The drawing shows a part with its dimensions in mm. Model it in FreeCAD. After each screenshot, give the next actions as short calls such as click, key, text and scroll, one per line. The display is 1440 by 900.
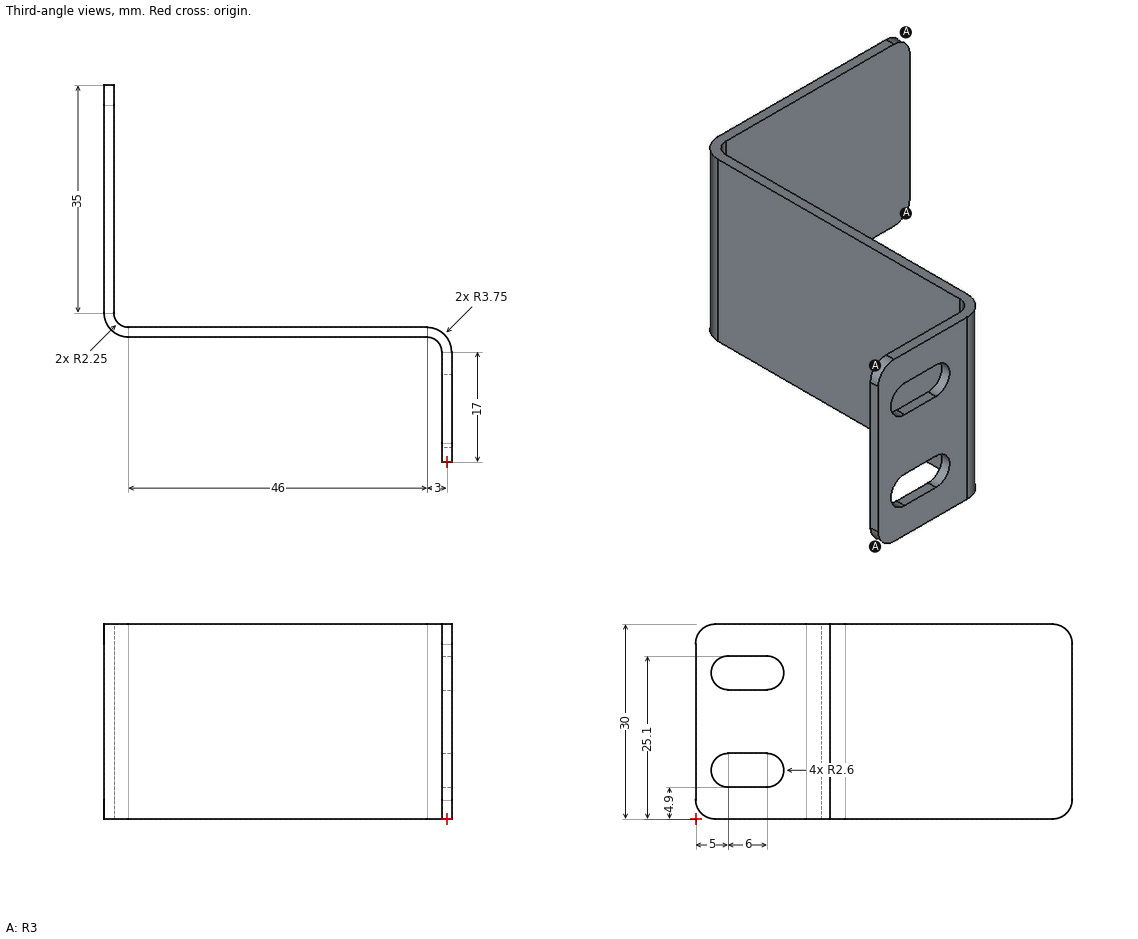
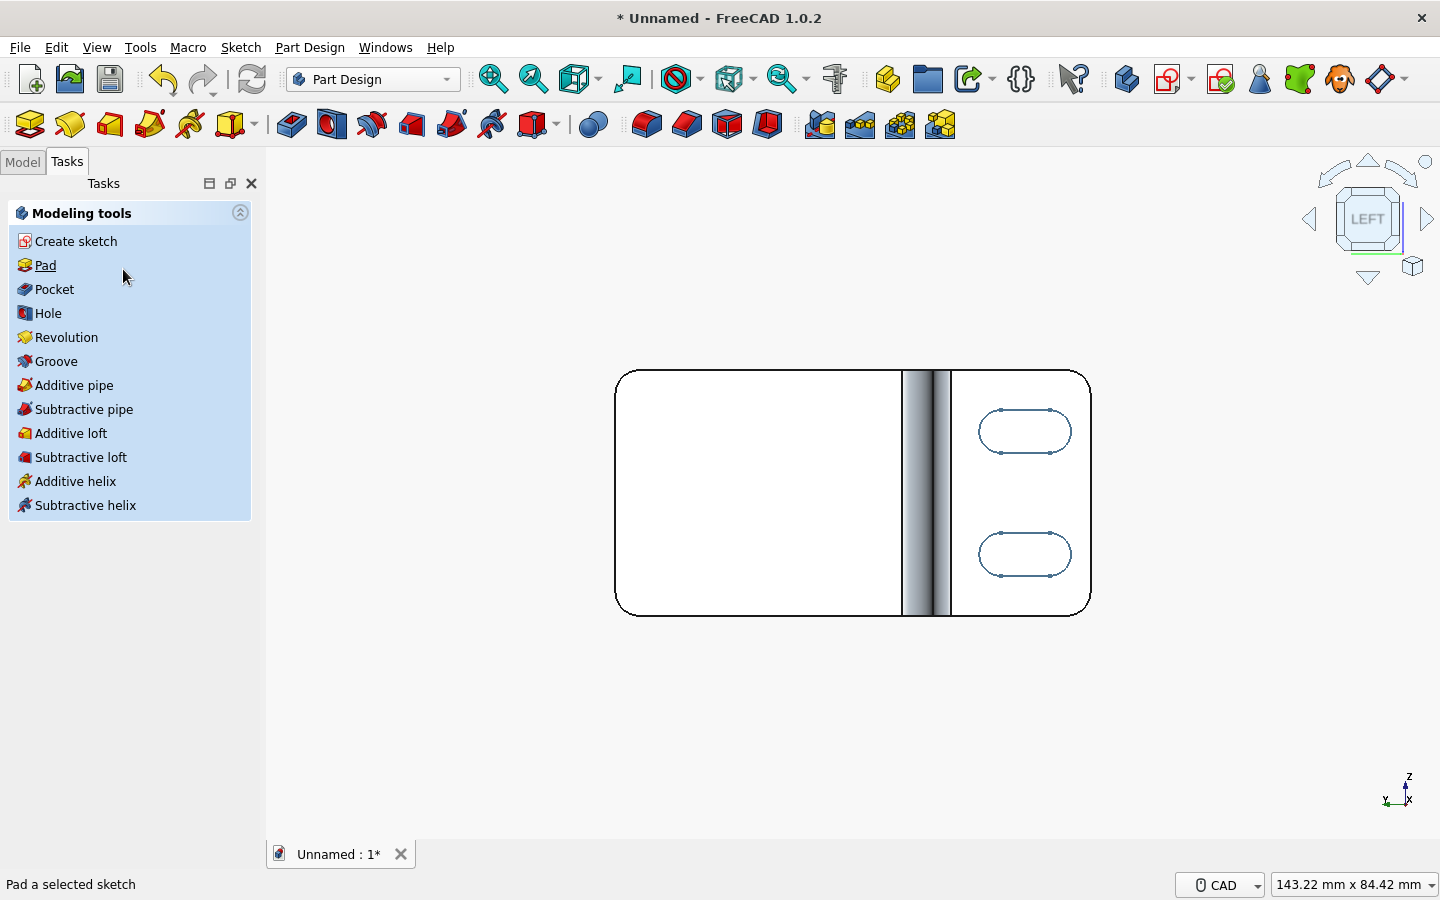
click(292, 124)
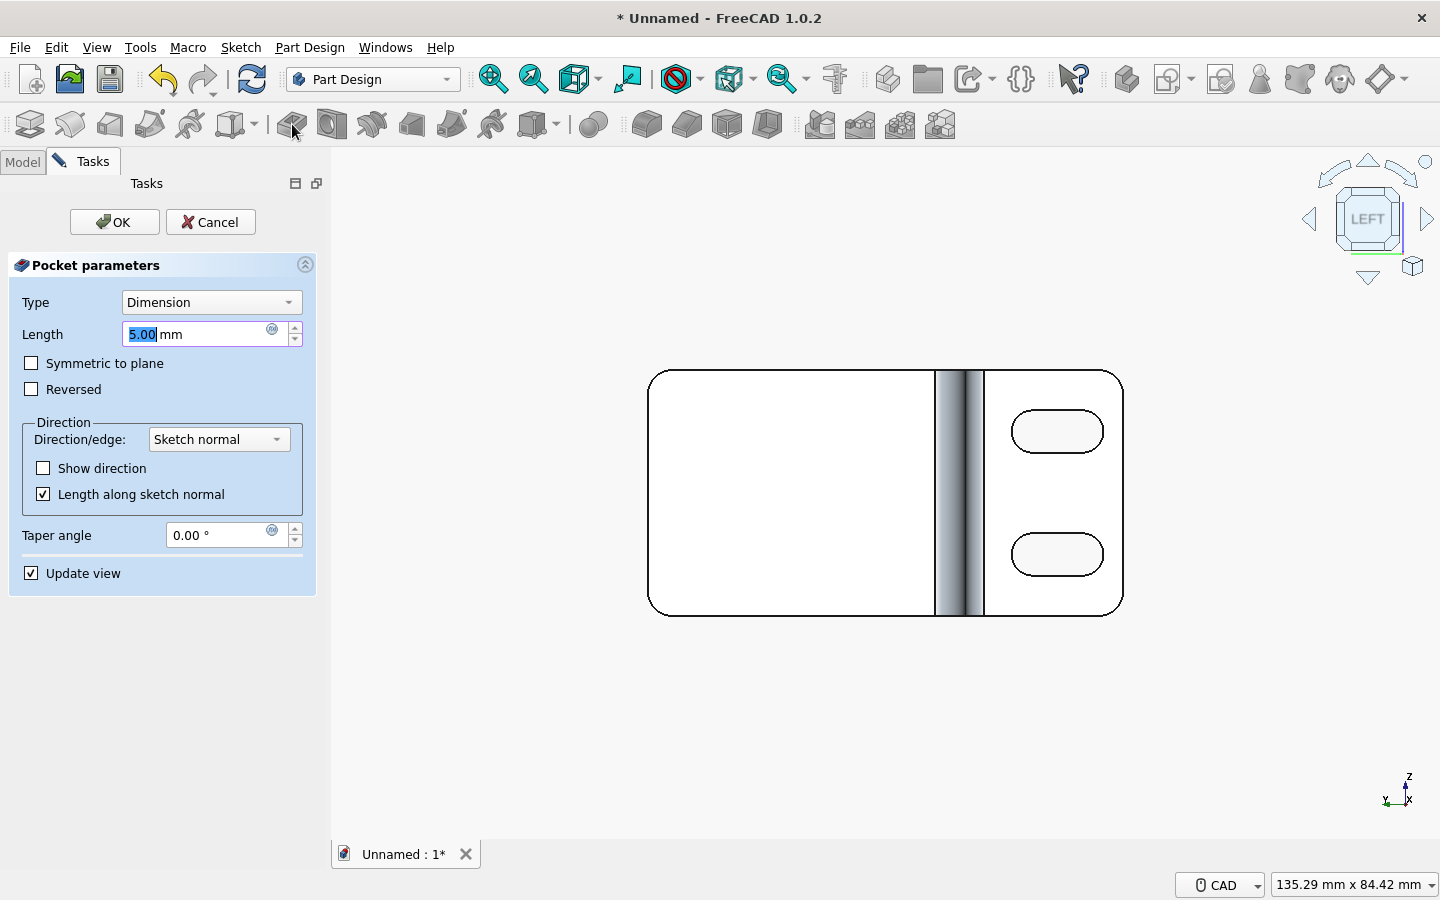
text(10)
key(Tab)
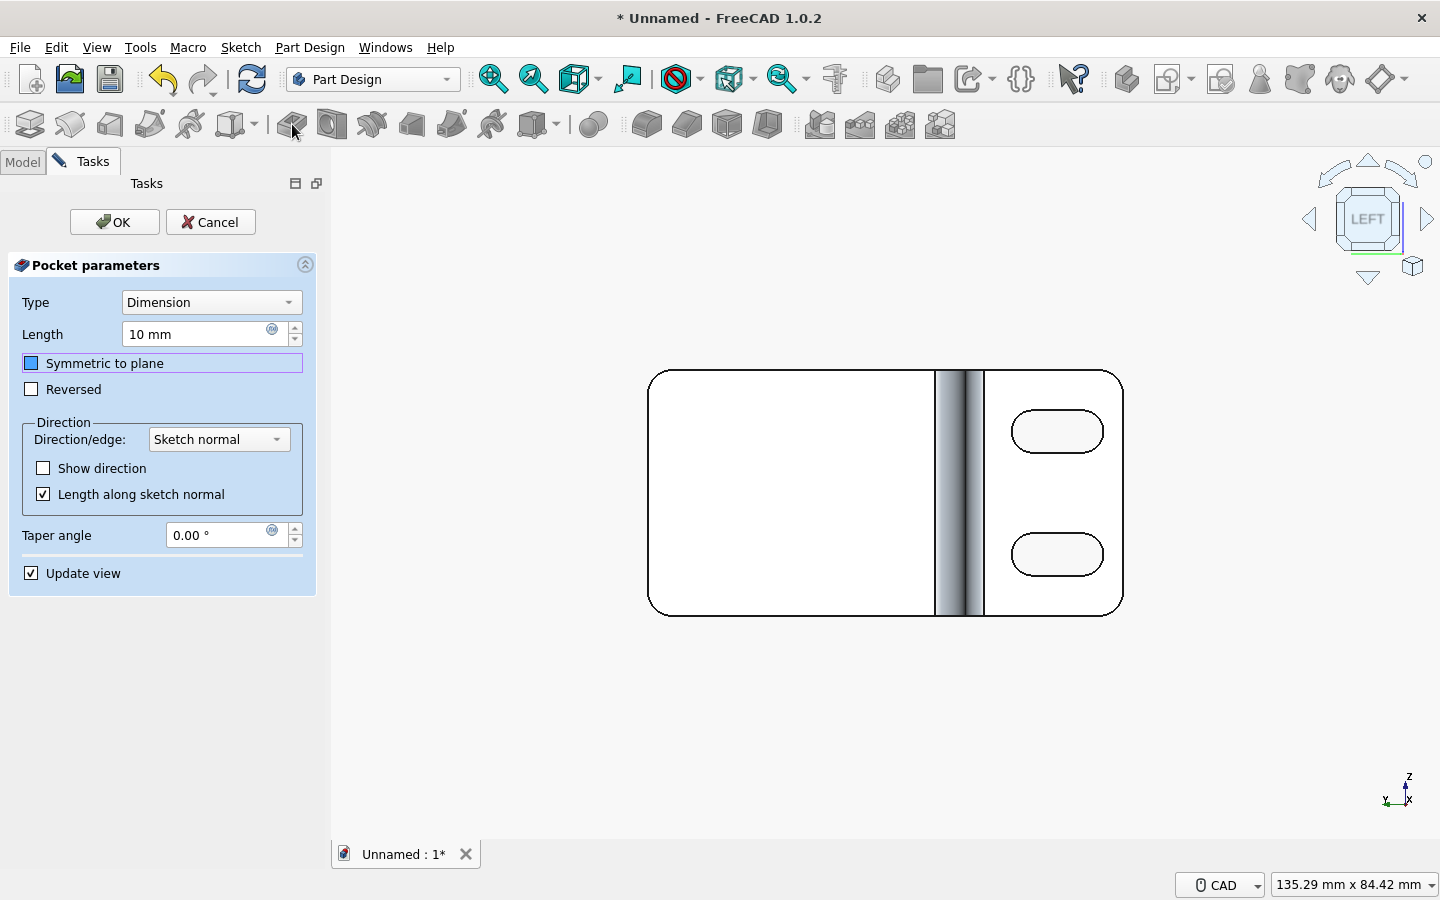
click(115, 222)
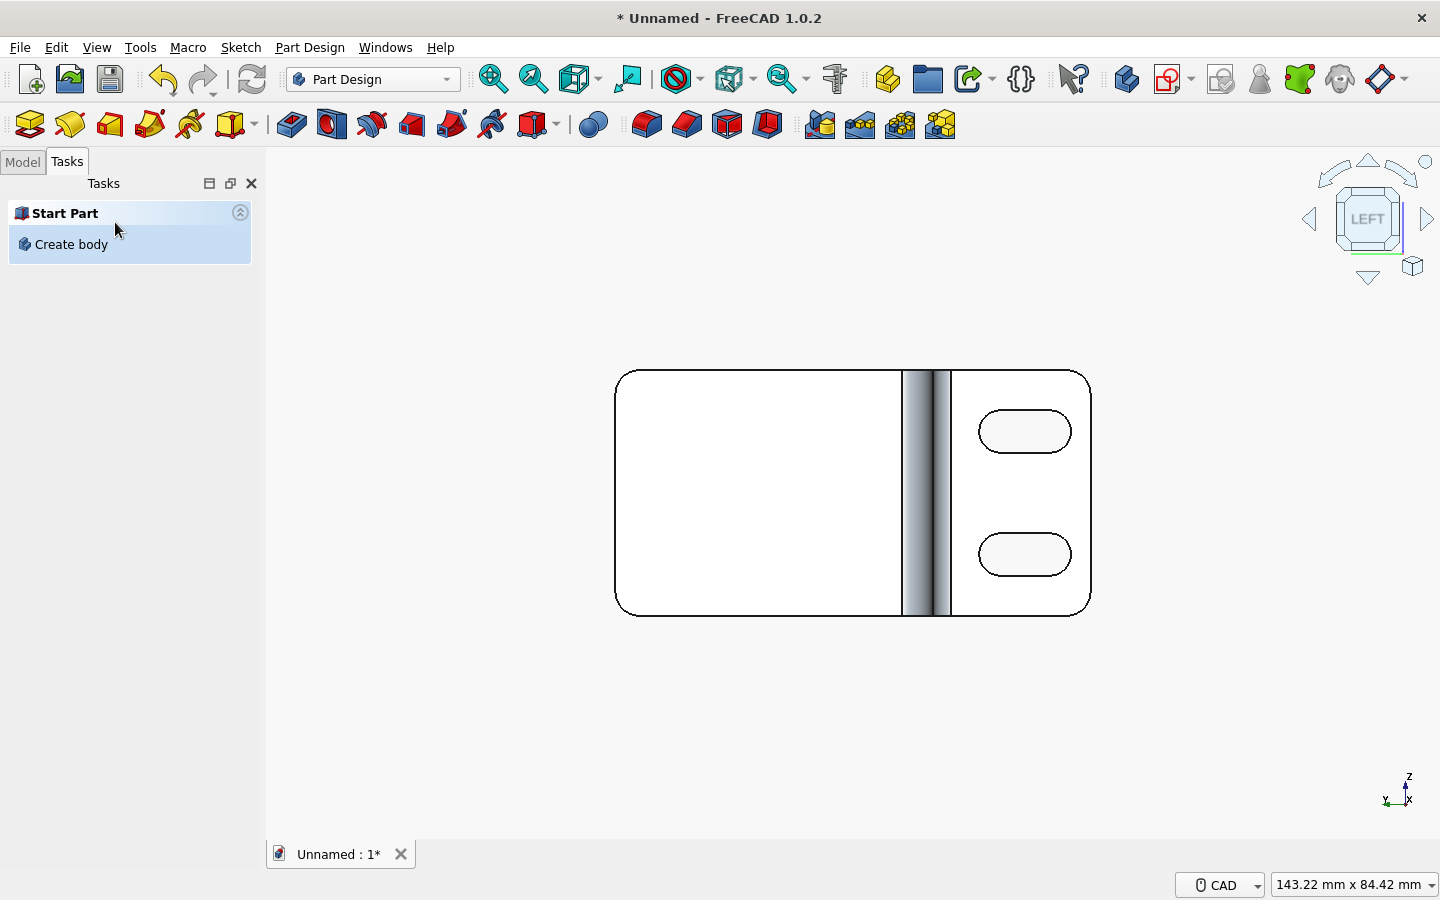
key(0)